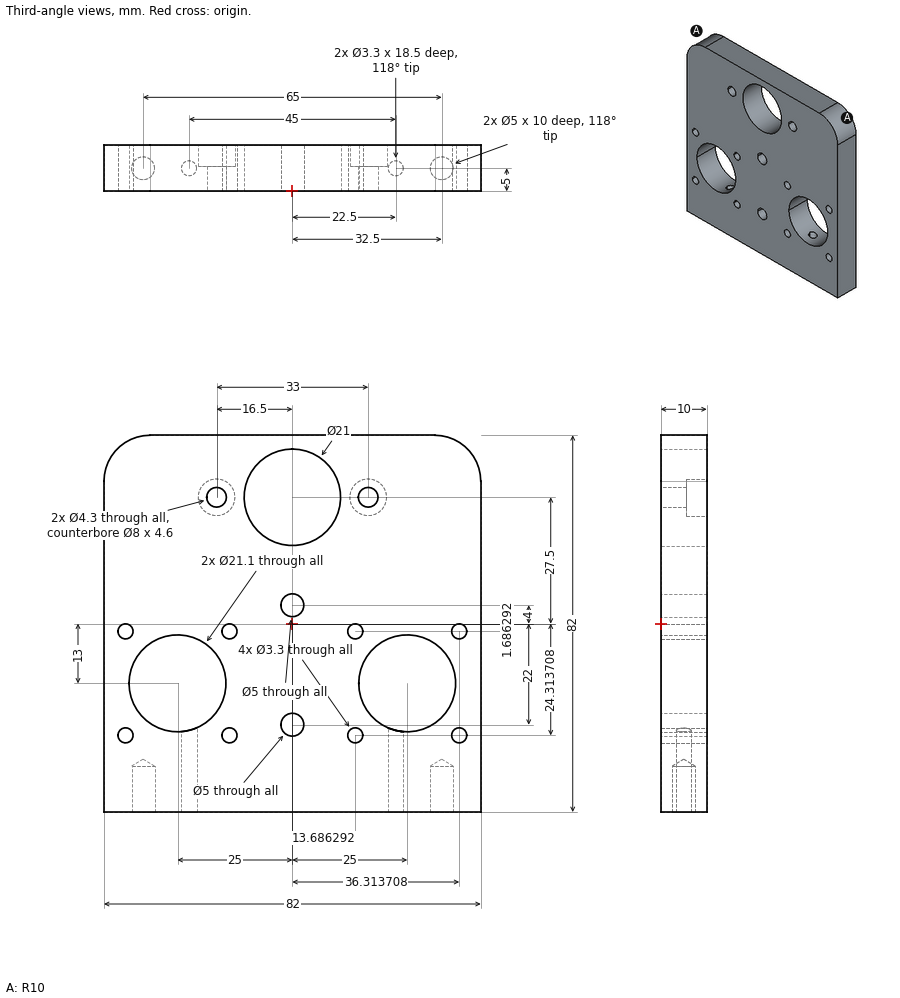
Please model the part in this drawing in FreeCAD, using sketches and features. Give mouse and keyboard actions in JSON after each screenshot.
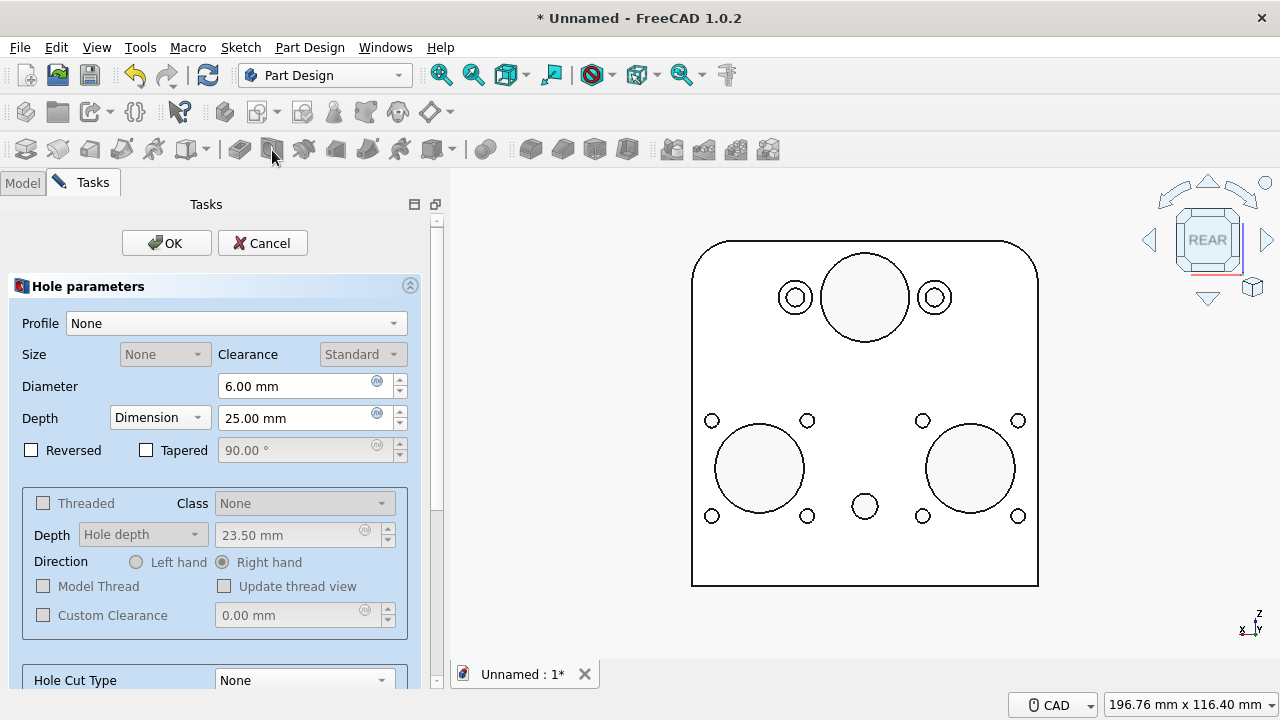
{"action": "triple_click", "coordinate": [305, 386]}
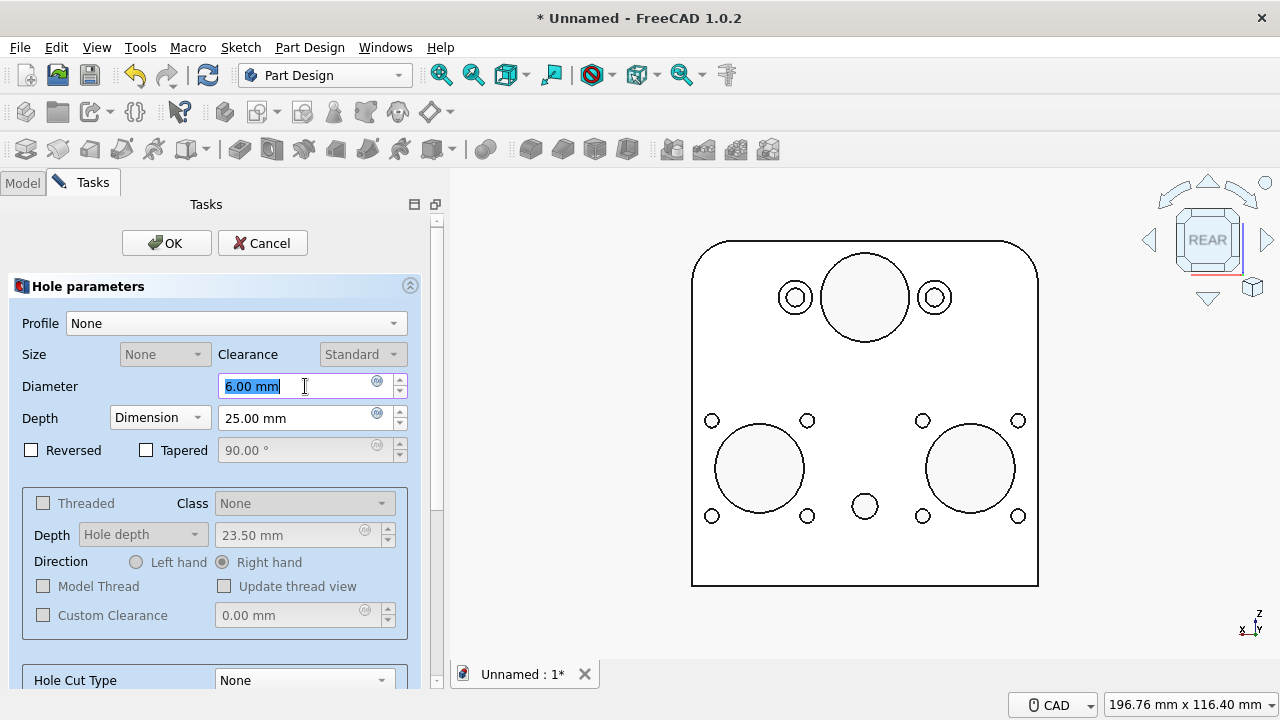
{"action": "type", "text": "5"}
{"action": "key", "text": "Tab"}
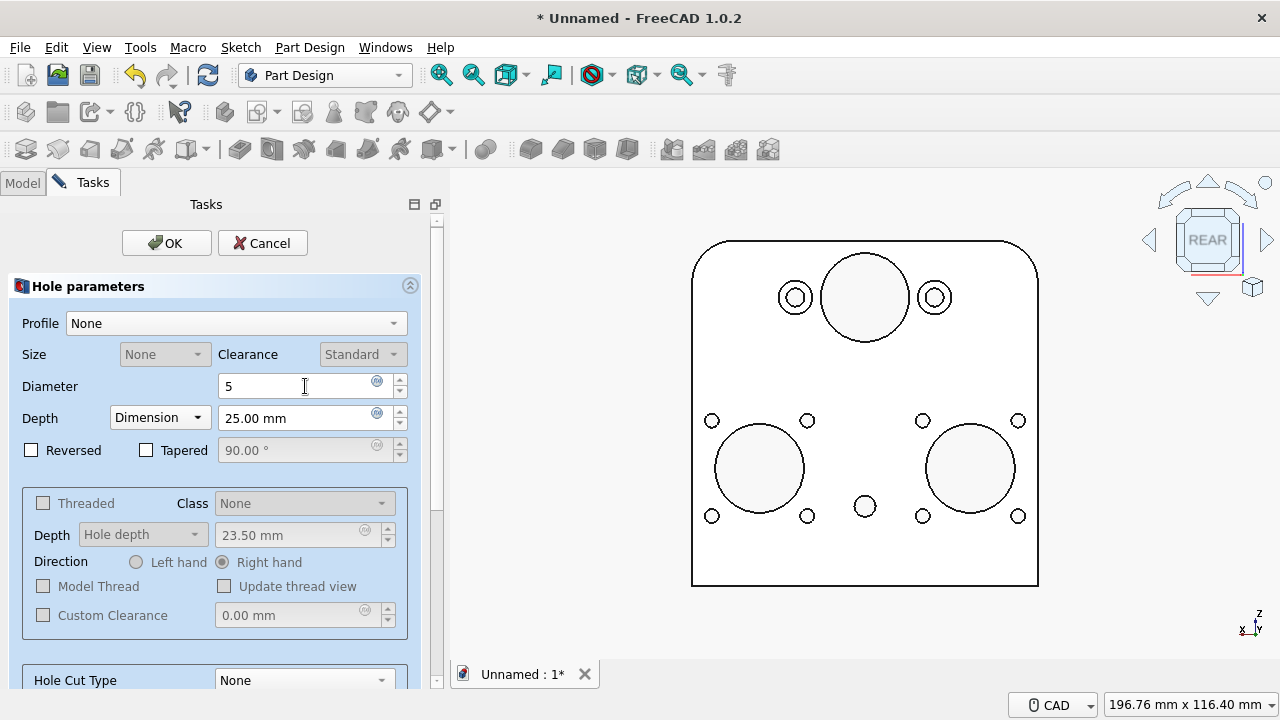
{"action": "left_click", "coordinate": [161, 418]}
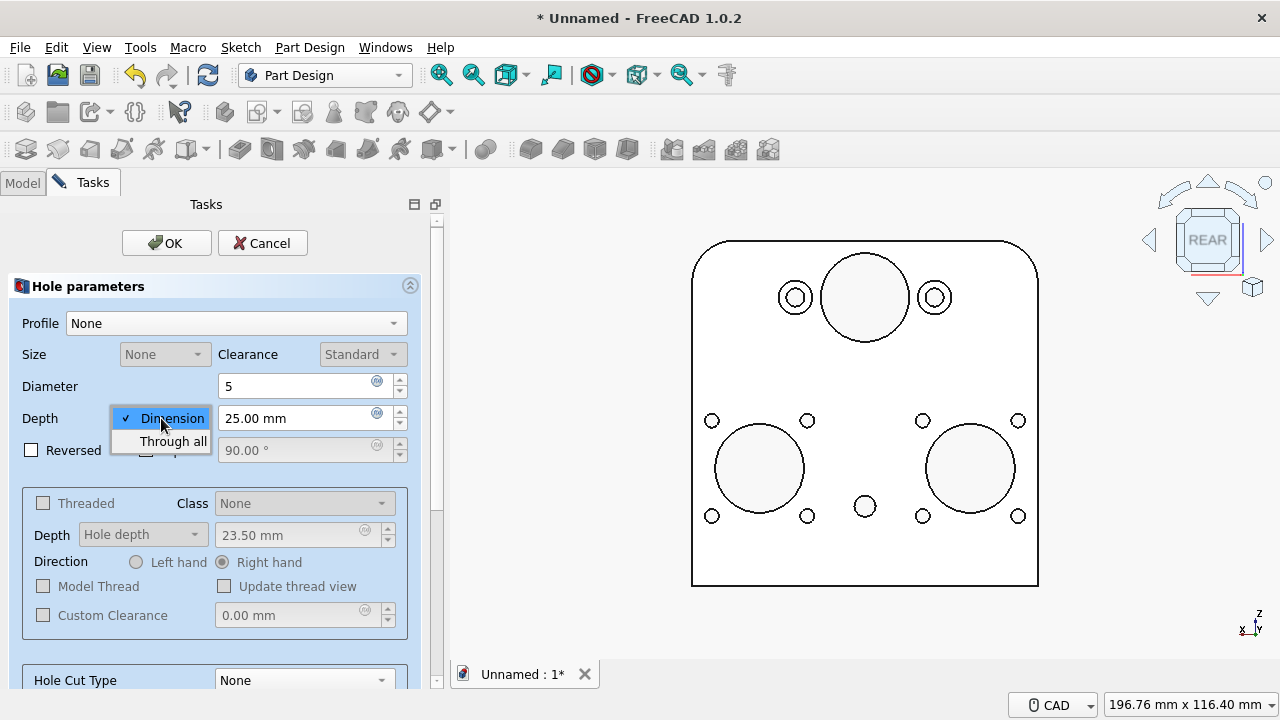
{"action": "left_click", "coordinate": [160, 442]}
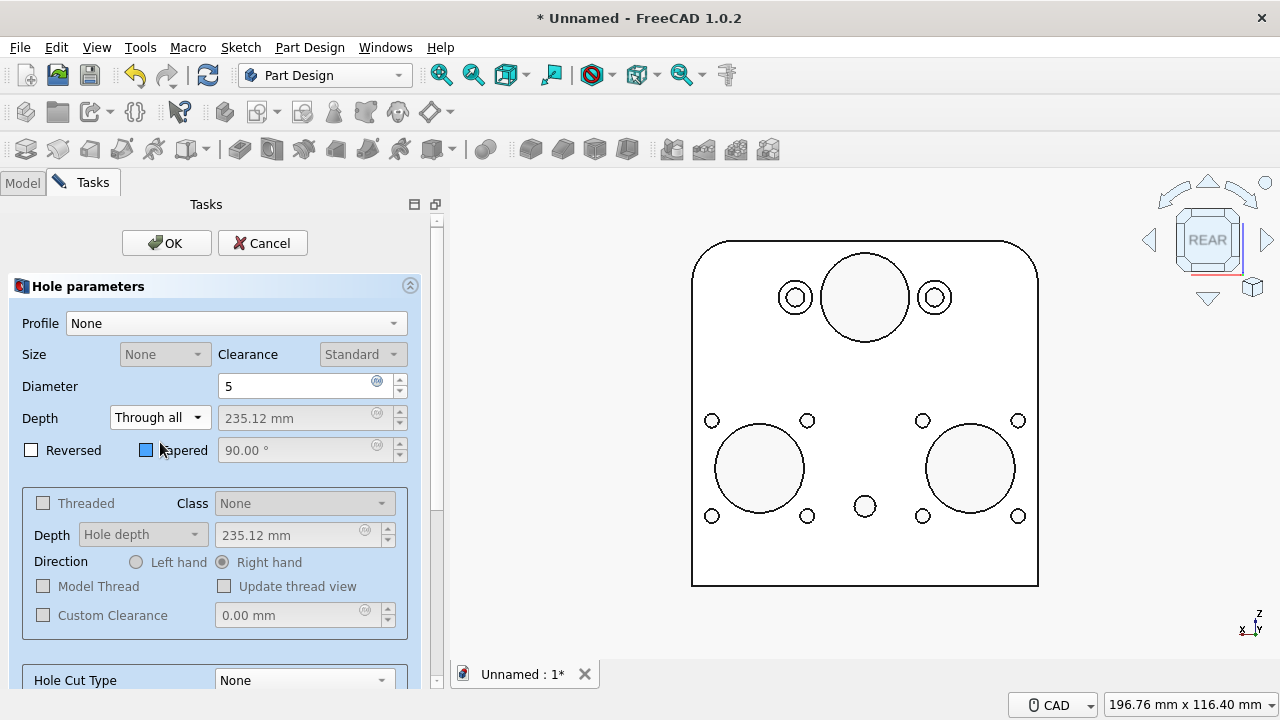
{"action": "left_click", "coordinate": [167, 243]}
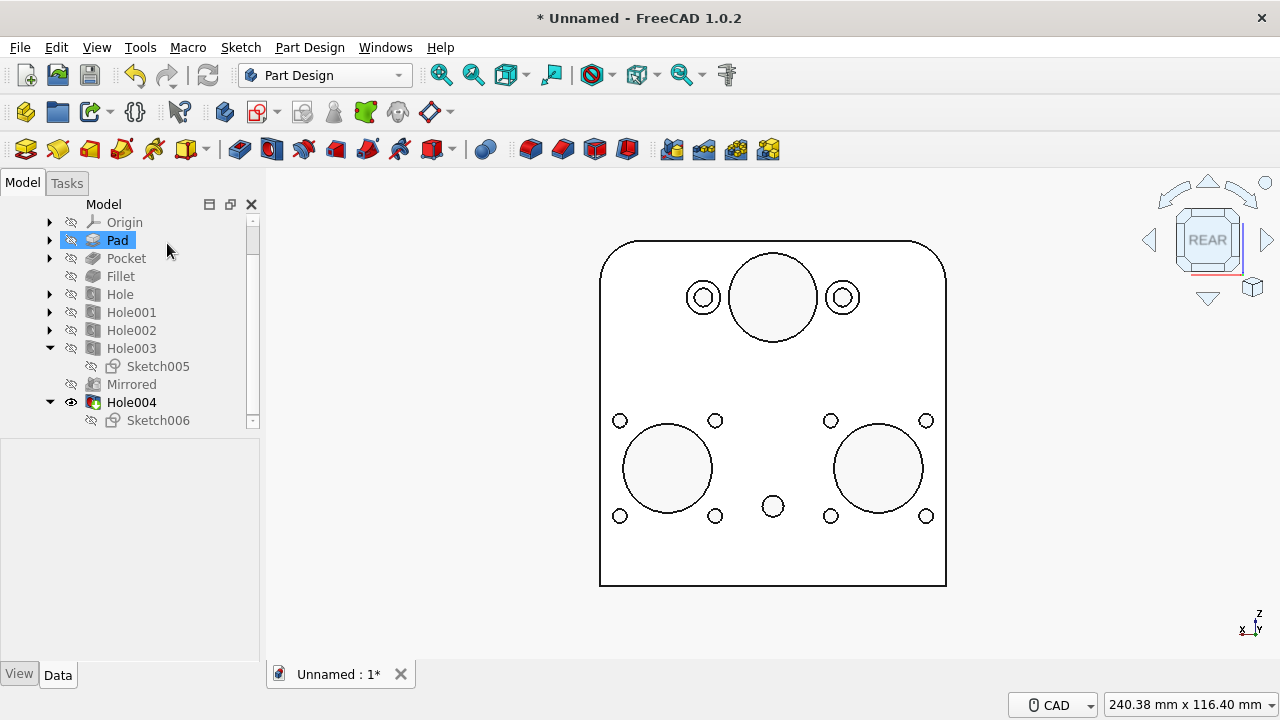
{"action": "left_click", "coordinate": [872, 363]}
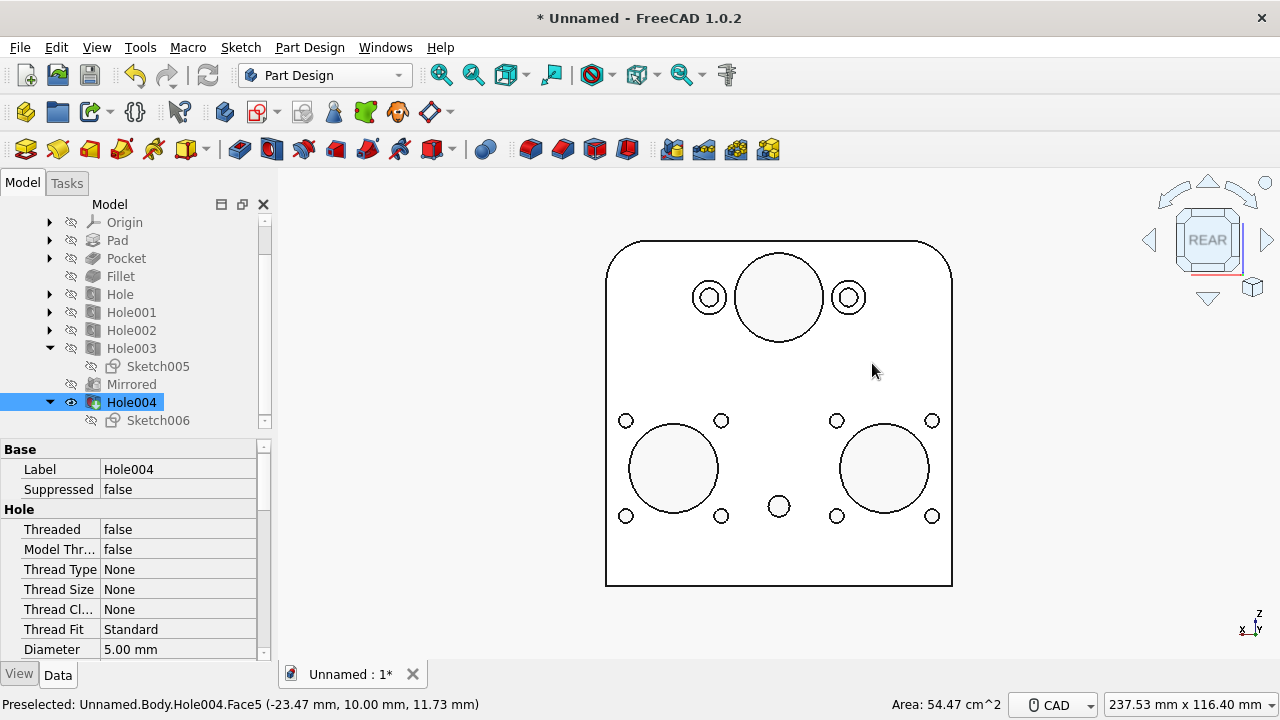
{"action": "left_click", "coordinate": [258, 112]}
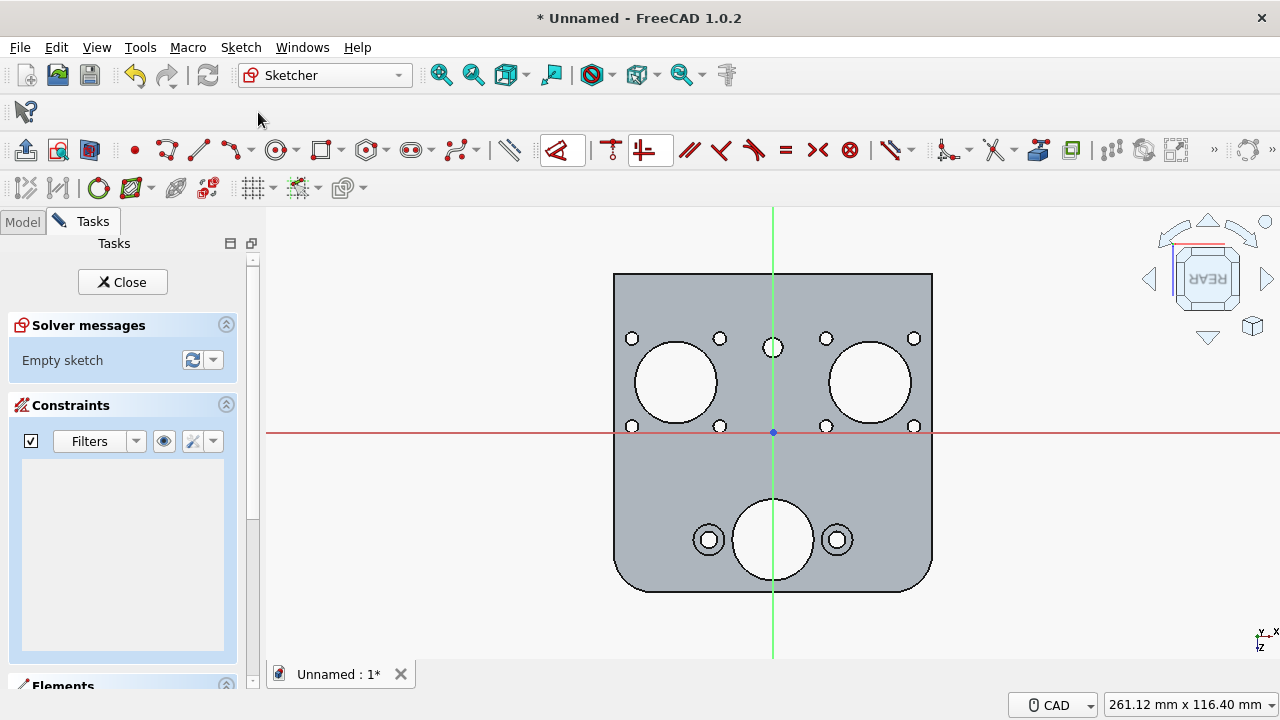
{"action": "scroll", "coordinate": [780, 447], "scroll_direction": "up", "scroll_amount": 12}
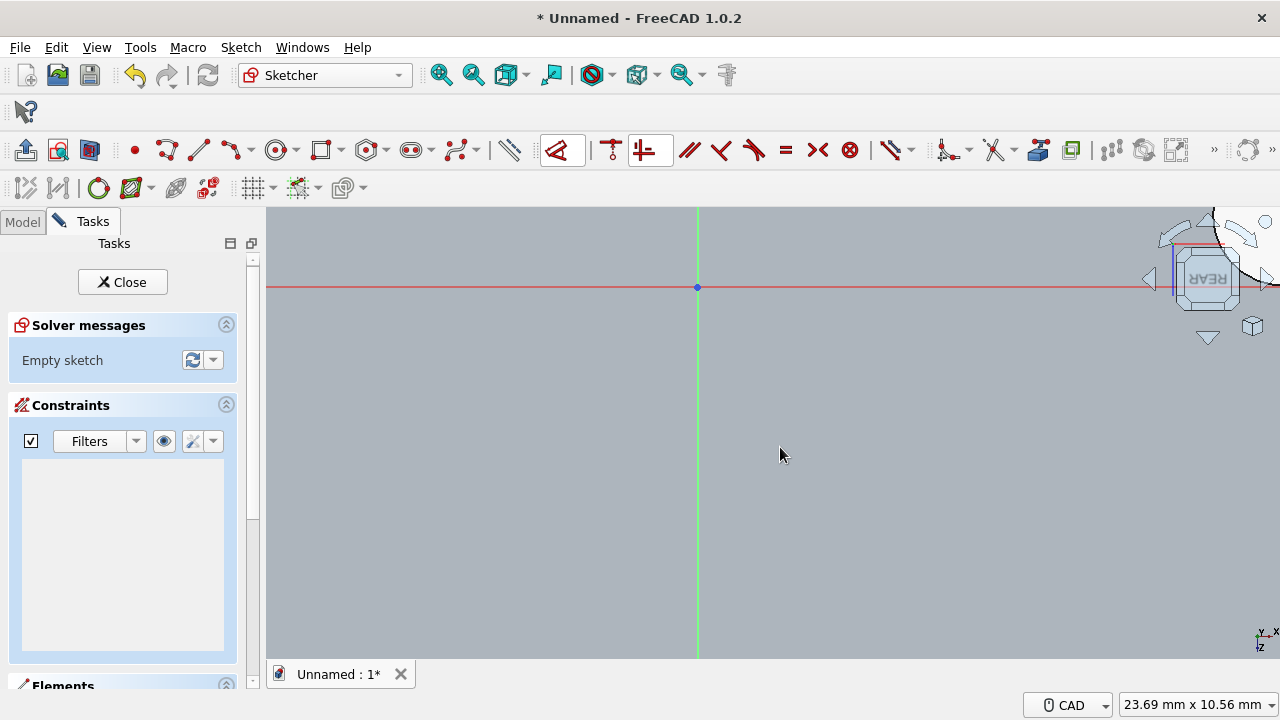
{"action": "left_click", "coordinate": [276, 150]}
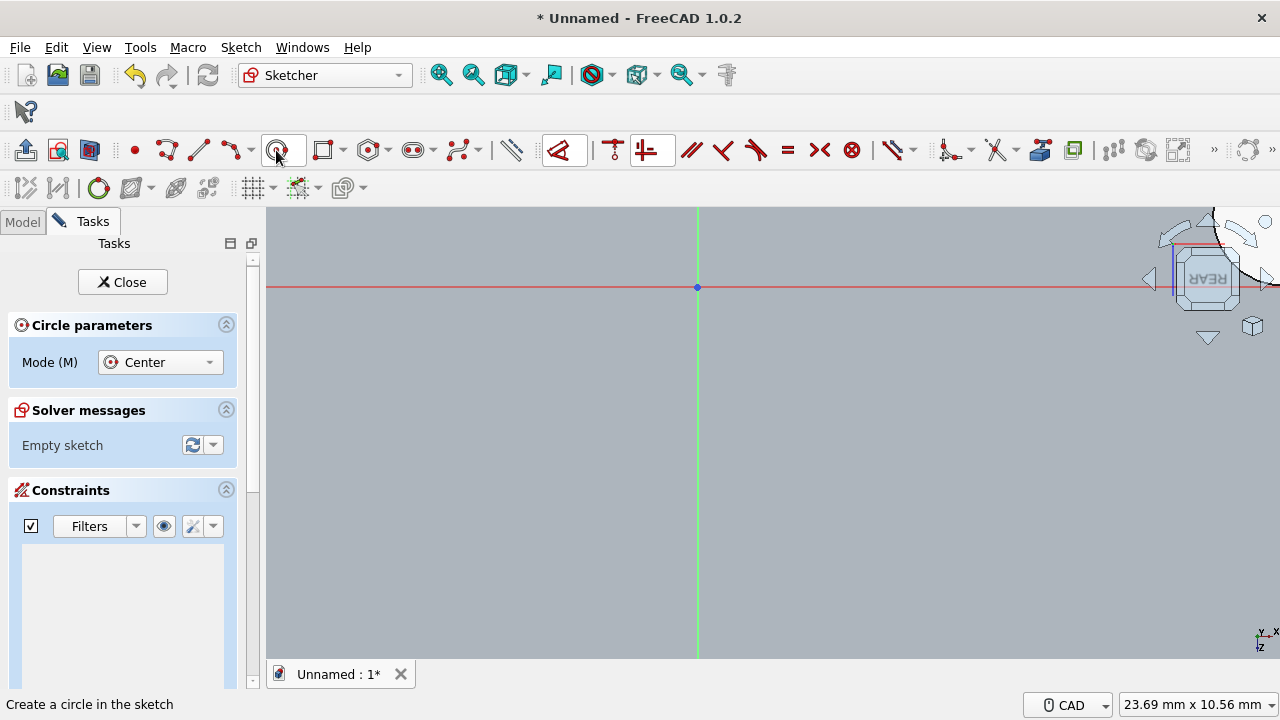
{"action": "left_click", "coordinate": [698, 459]}
{"action": "left_click", "coordinate": [773, 383]}
{"action": "key", "text": "Escape"}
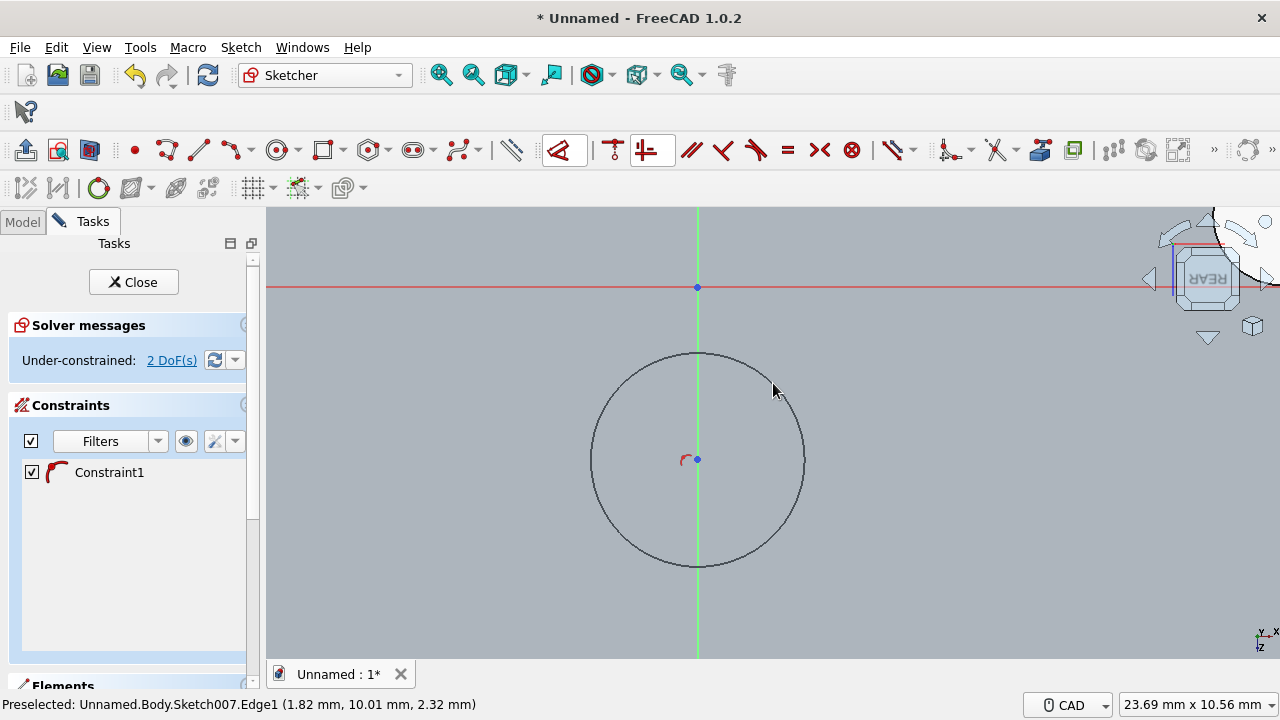
{"action": "left_click", "coordinate": [773, 384]}